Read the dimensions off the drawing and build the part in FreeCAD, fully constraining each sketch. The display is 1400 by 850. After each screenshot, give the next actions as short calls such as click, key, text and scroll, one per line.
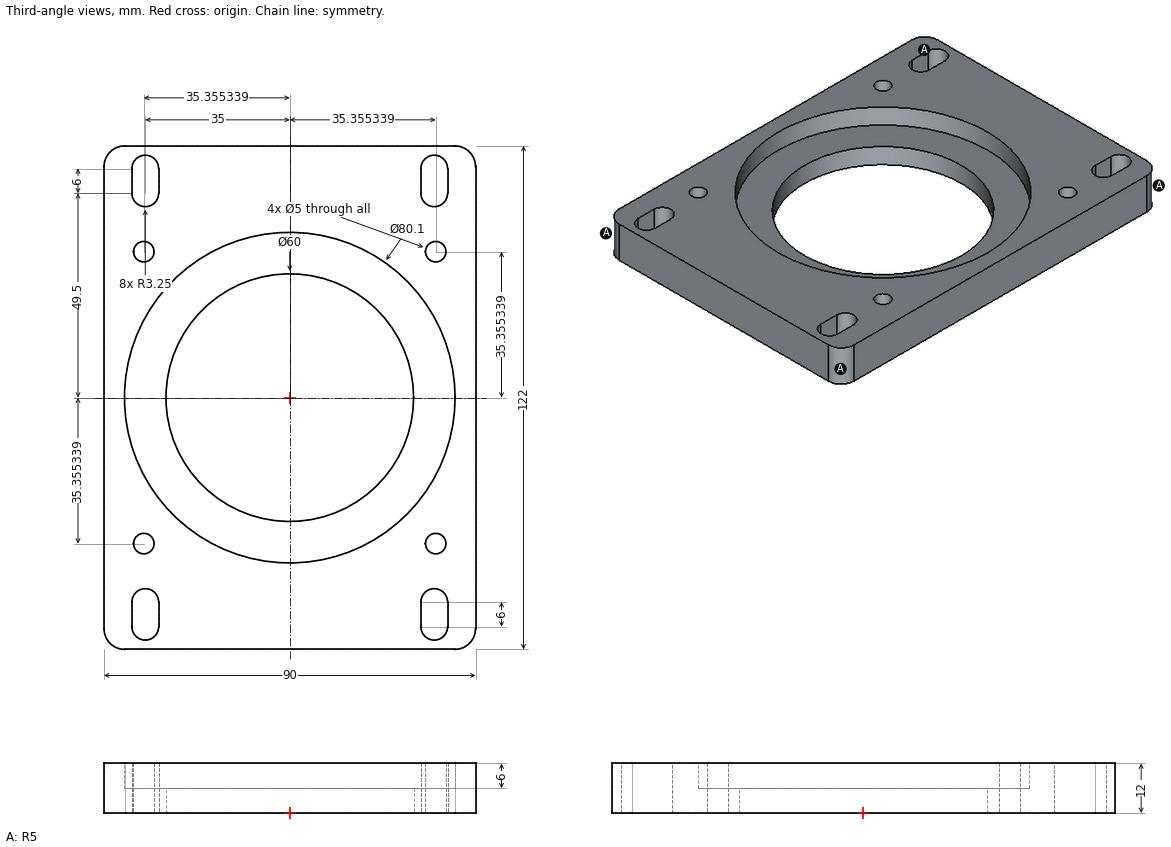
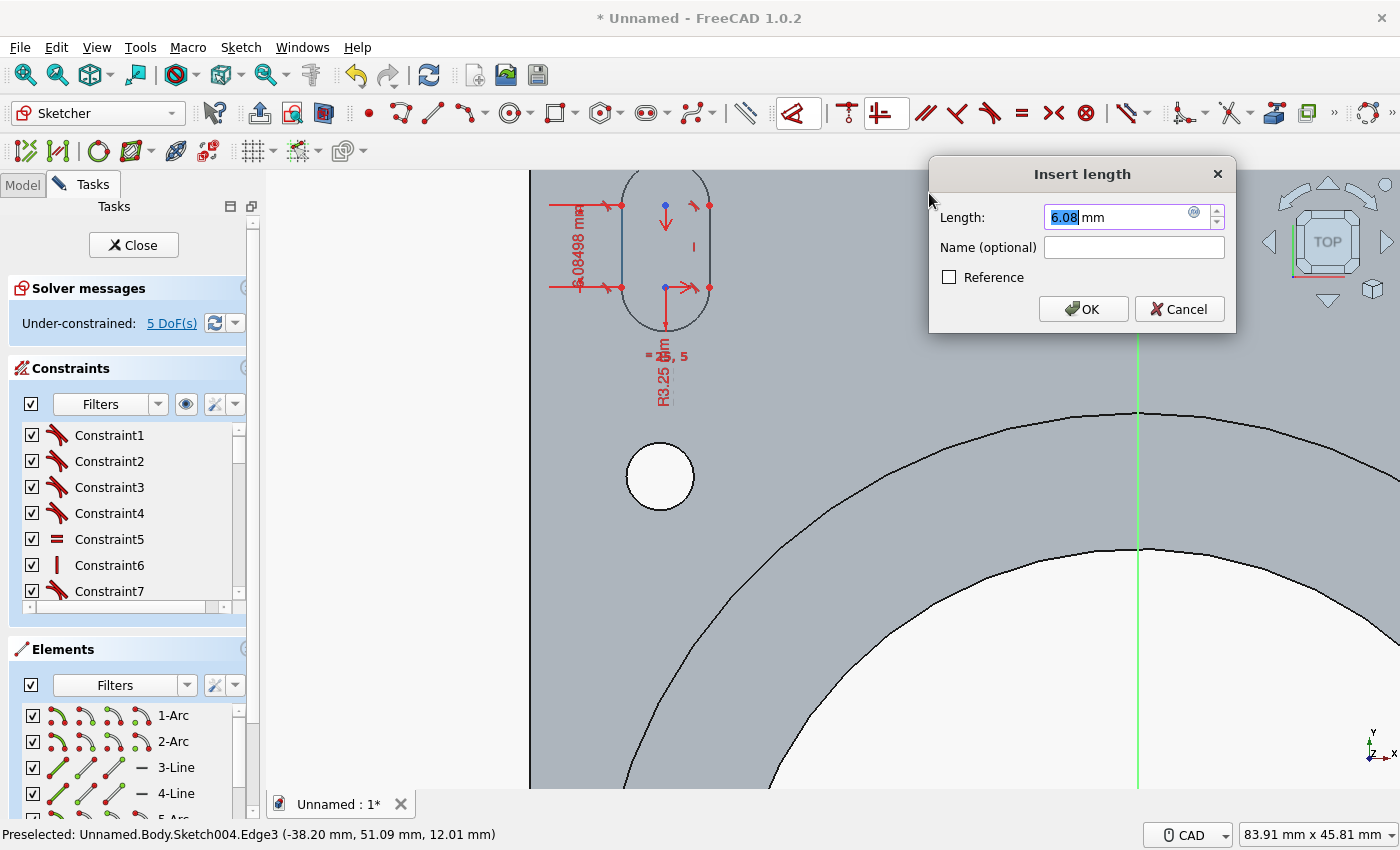
text(6)
key(Return)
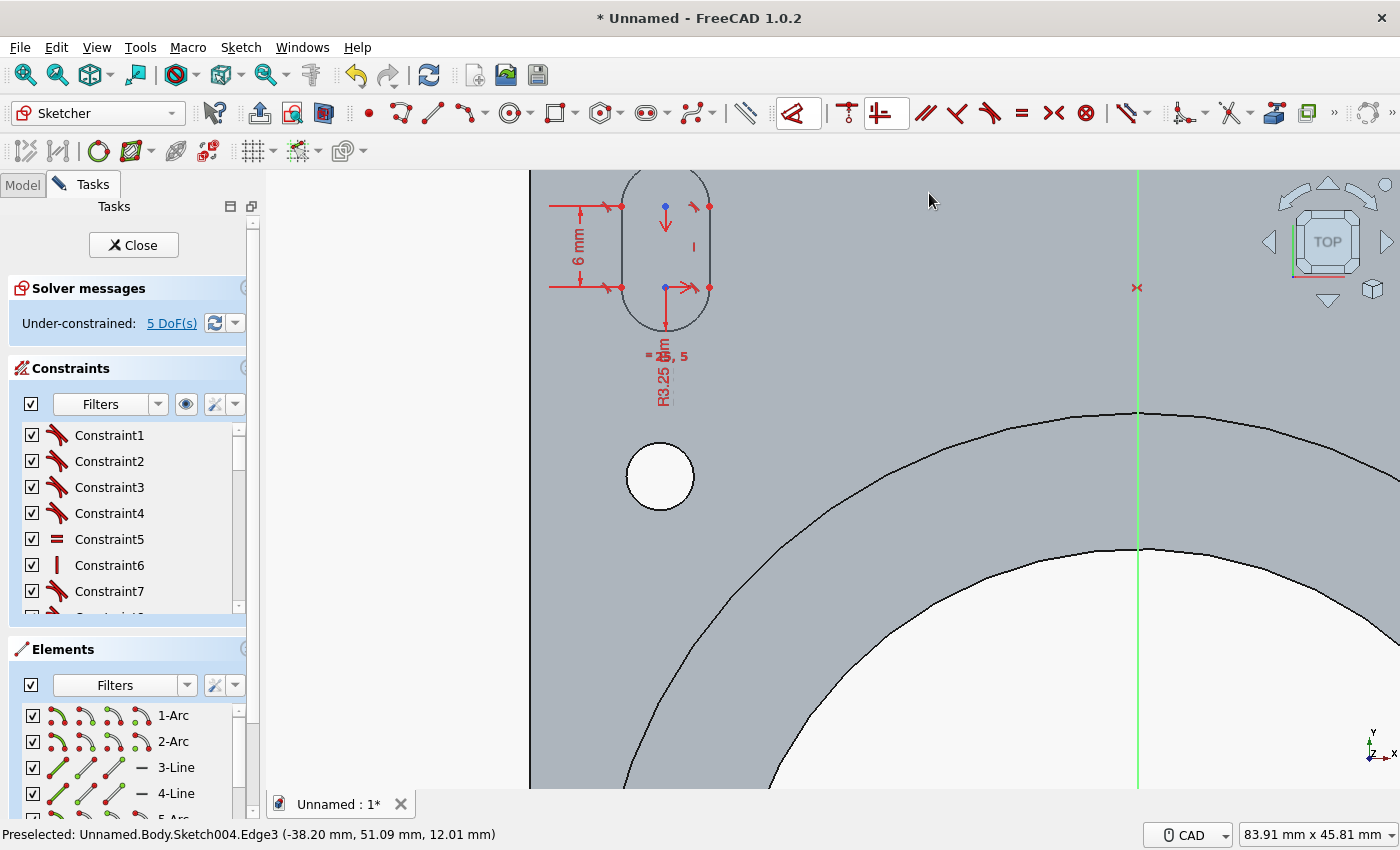
scroll(642, 324, down, 7)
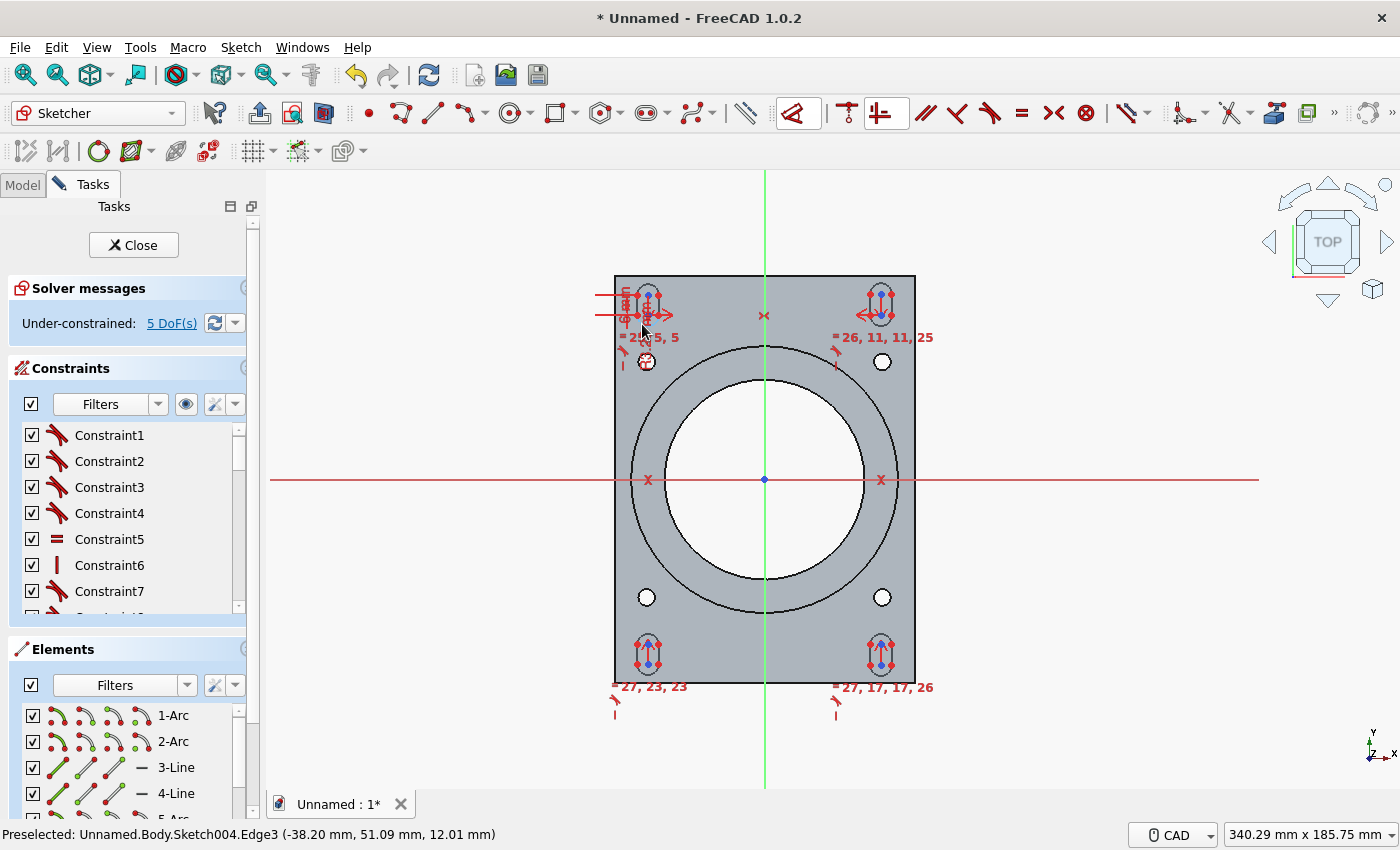
scroll(870, 309, up, 4)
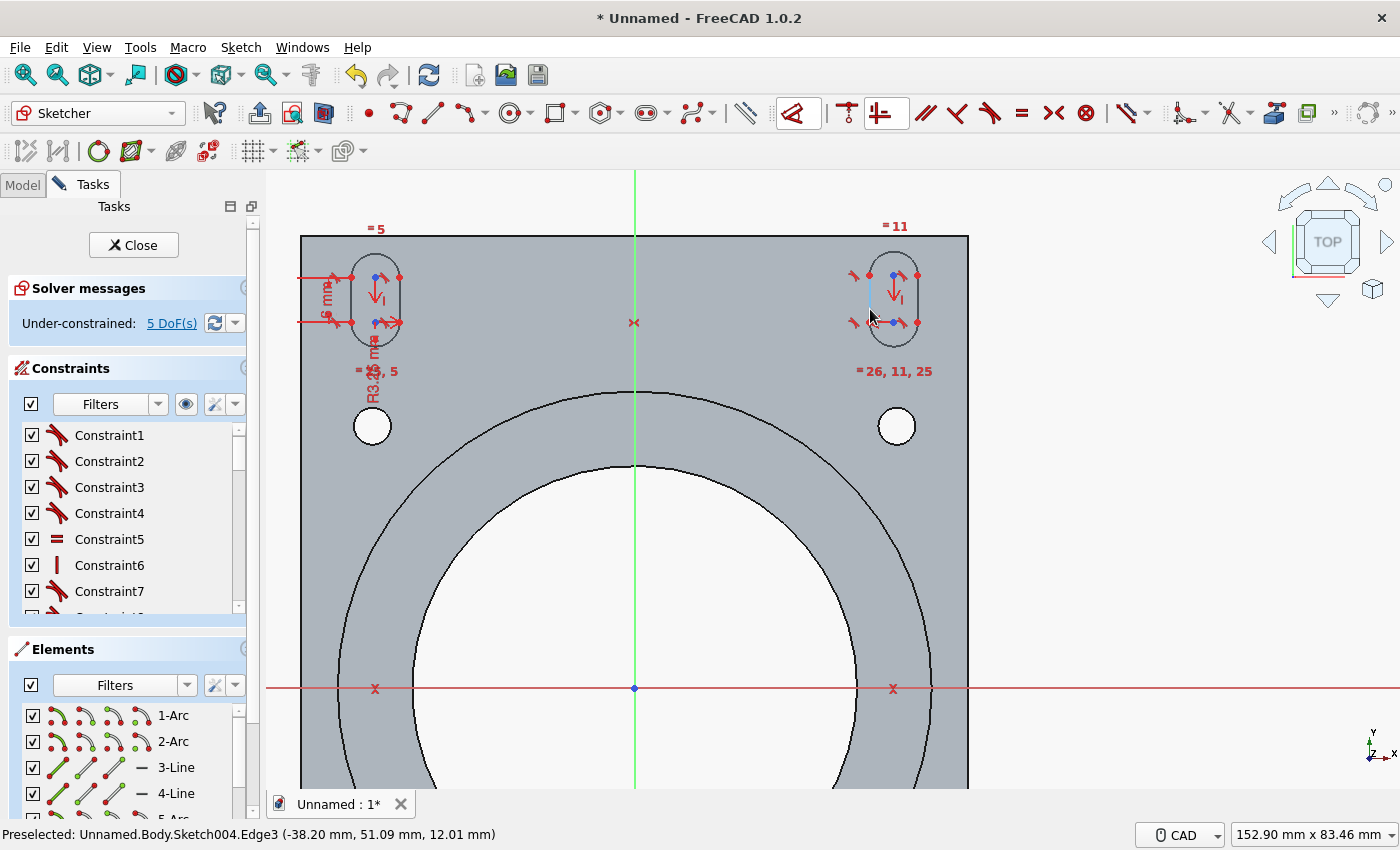
click(870, 308)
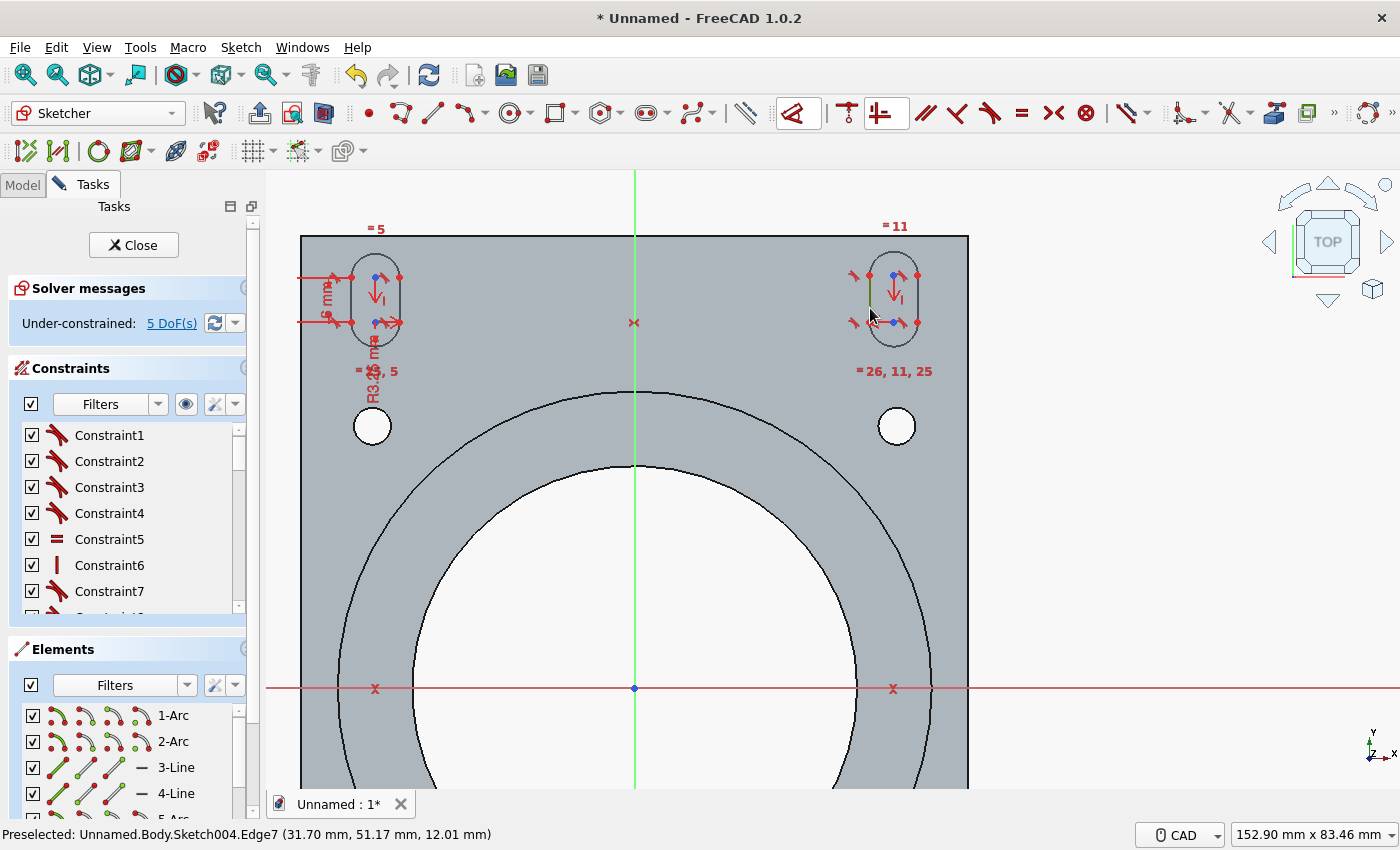
click(816, 114)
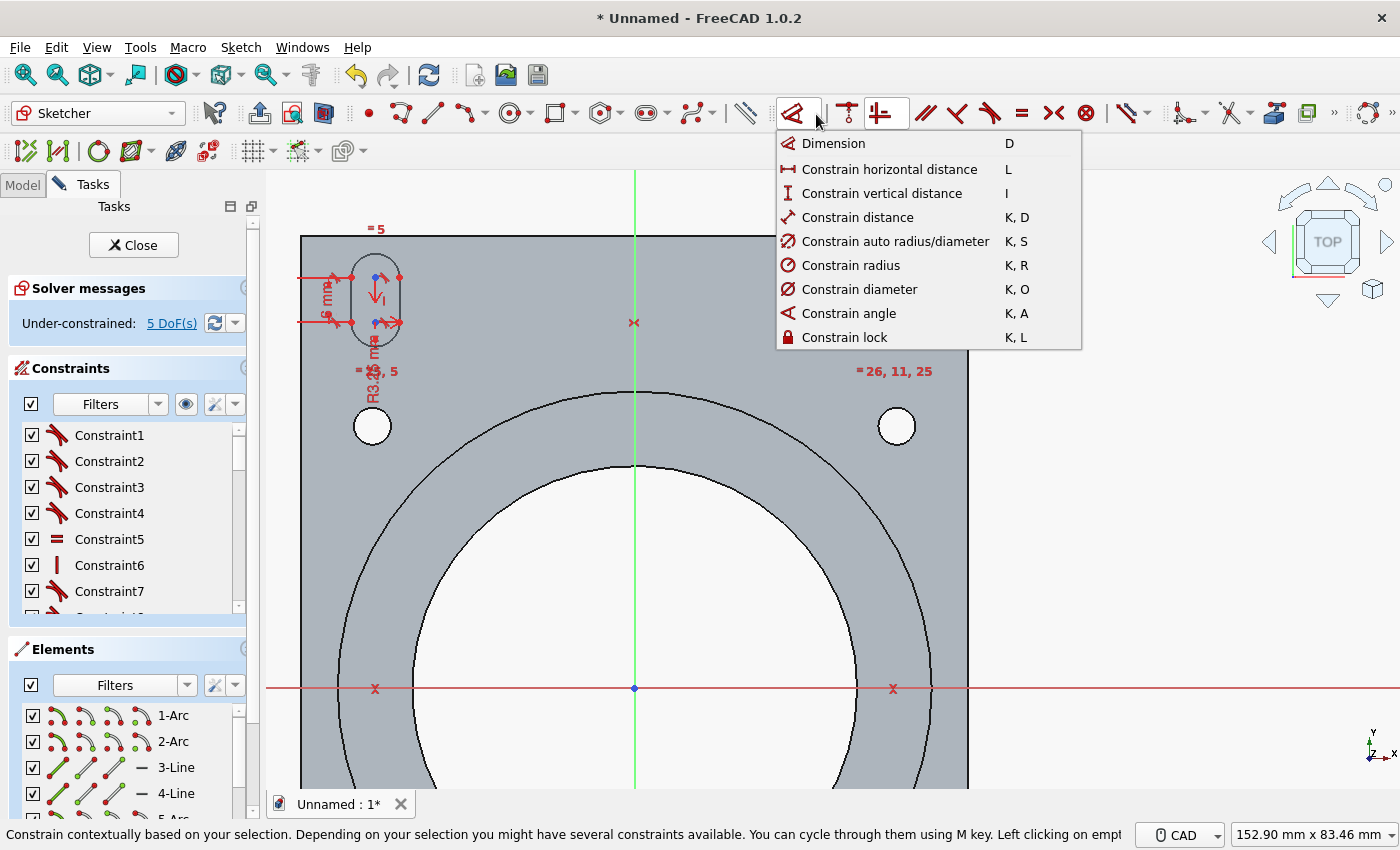
click(929, 193)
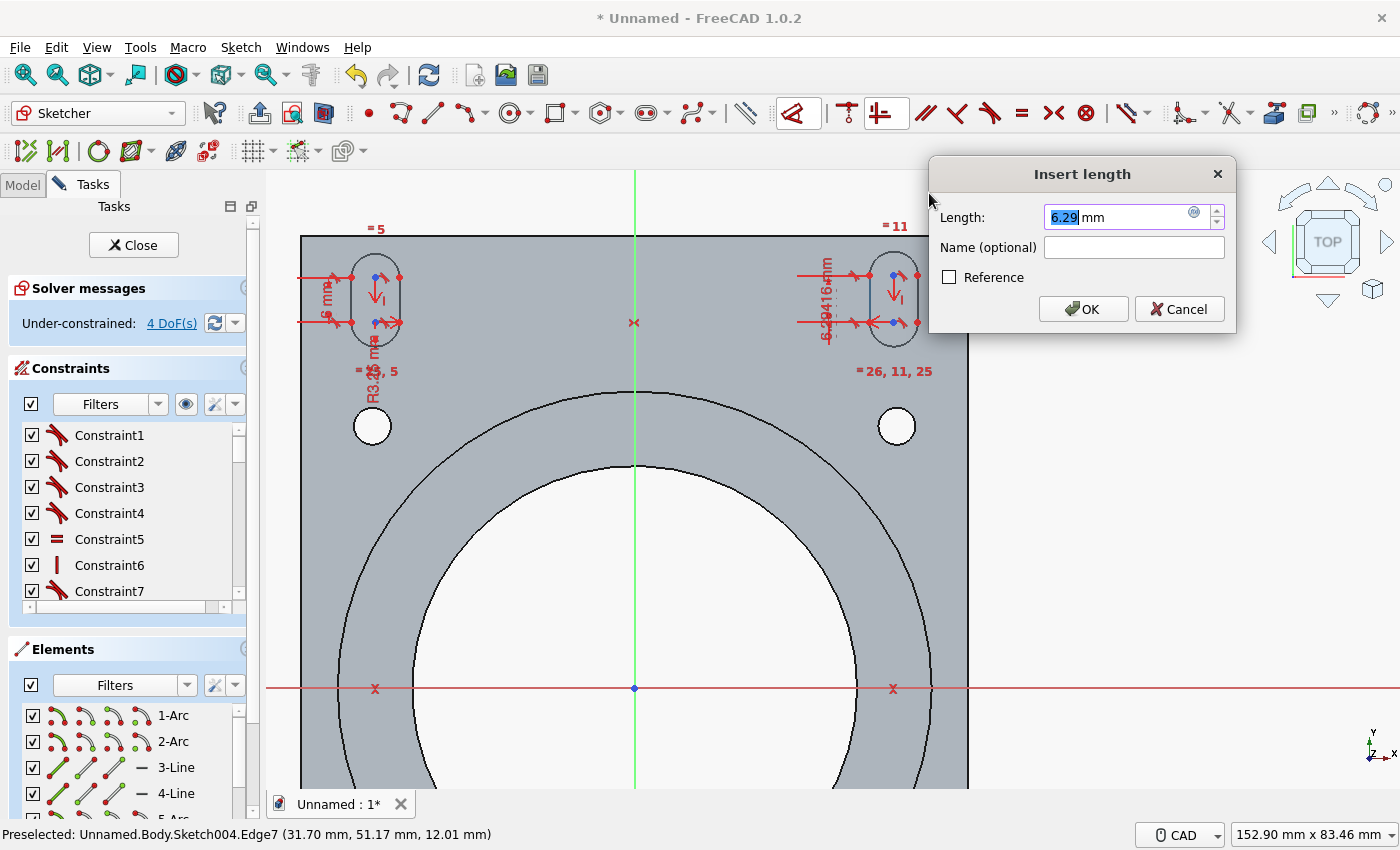
text(6)
key(Return)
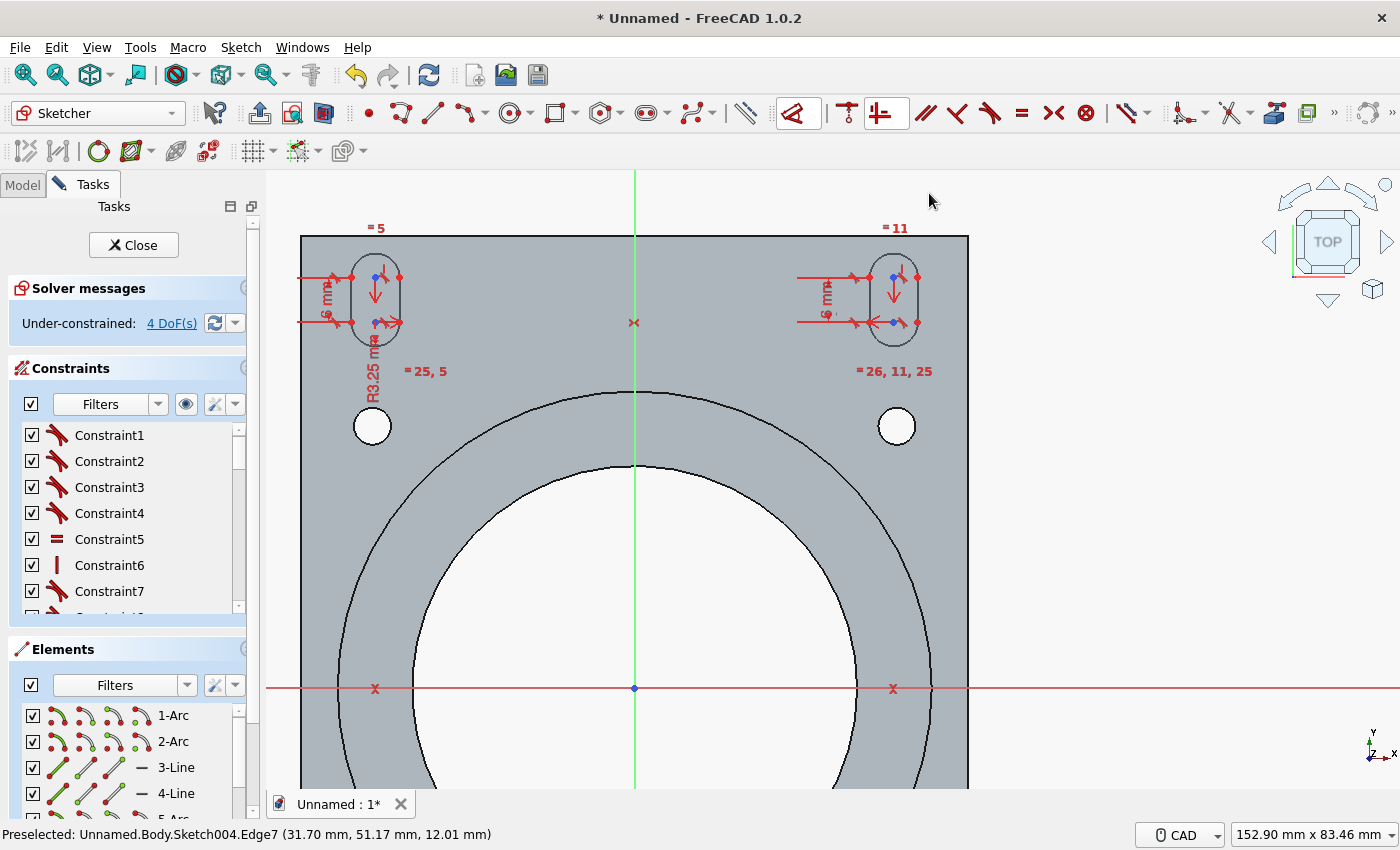
scroll(870, 309, down, 4)